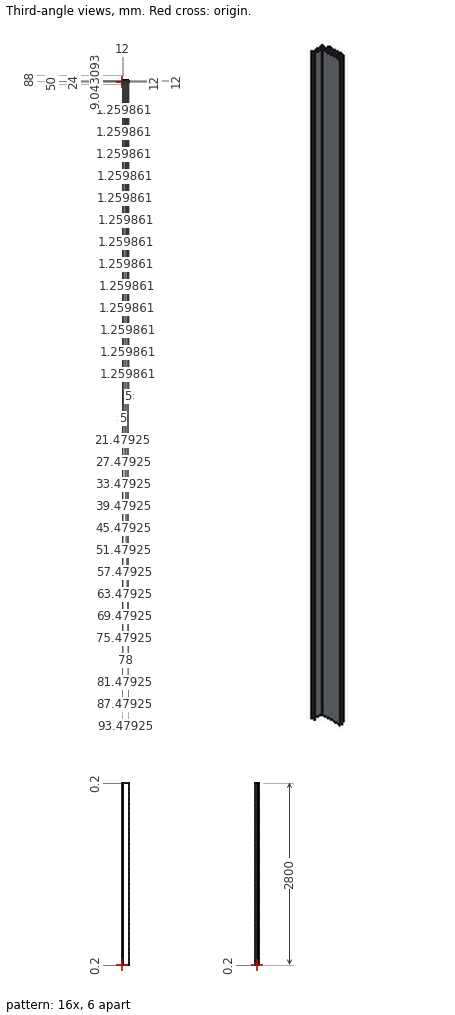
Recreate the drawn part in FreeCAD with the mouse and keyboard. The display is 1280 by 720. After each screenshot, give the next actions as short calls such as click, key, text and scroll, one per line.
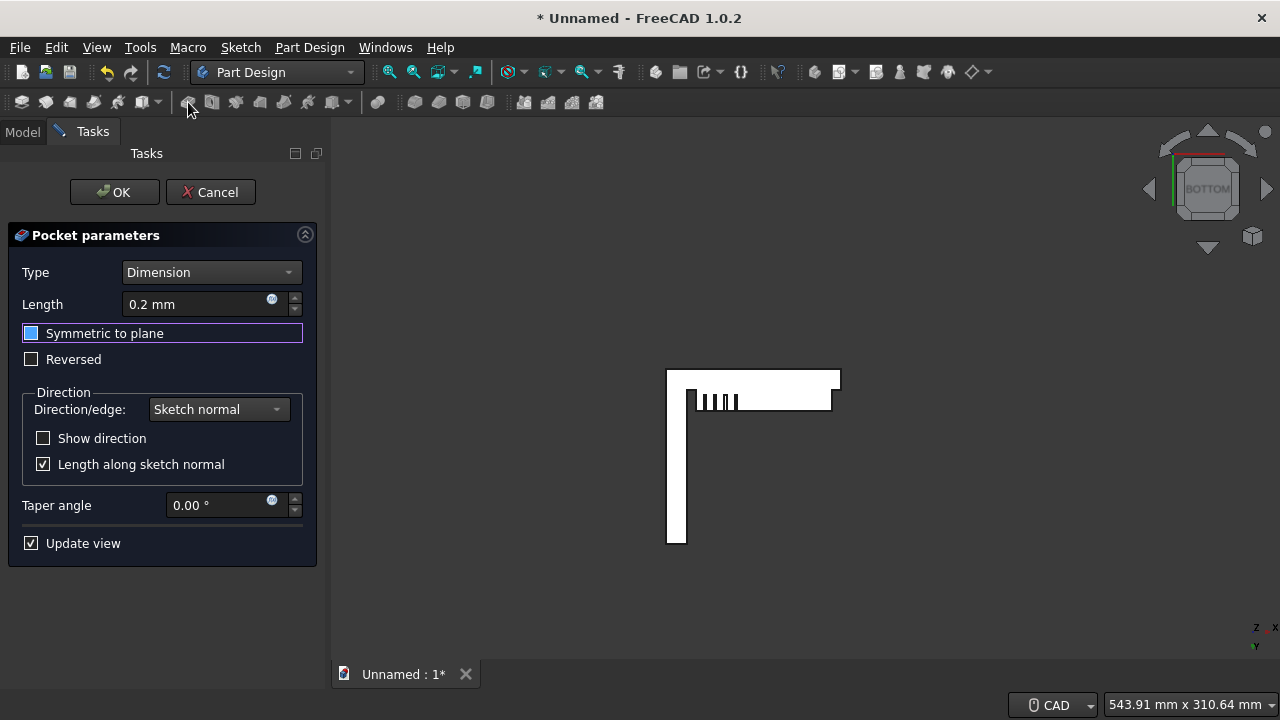
click(115, 192)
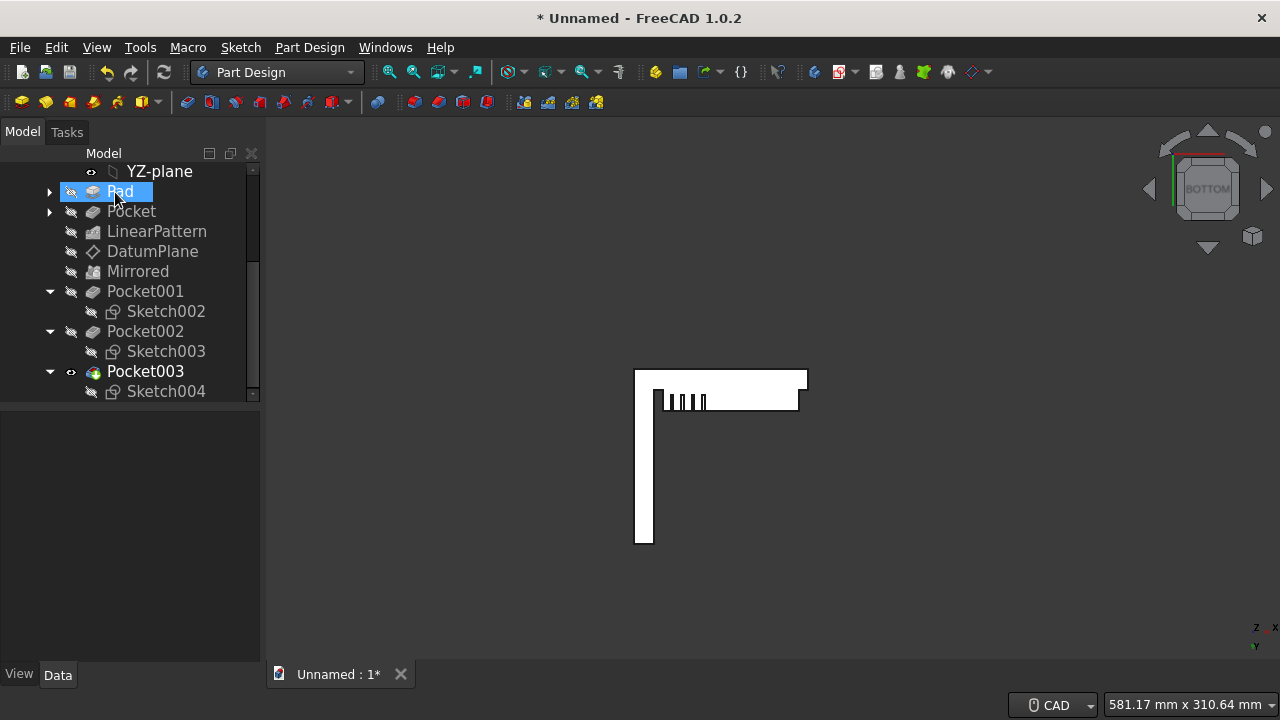
click(390, 72)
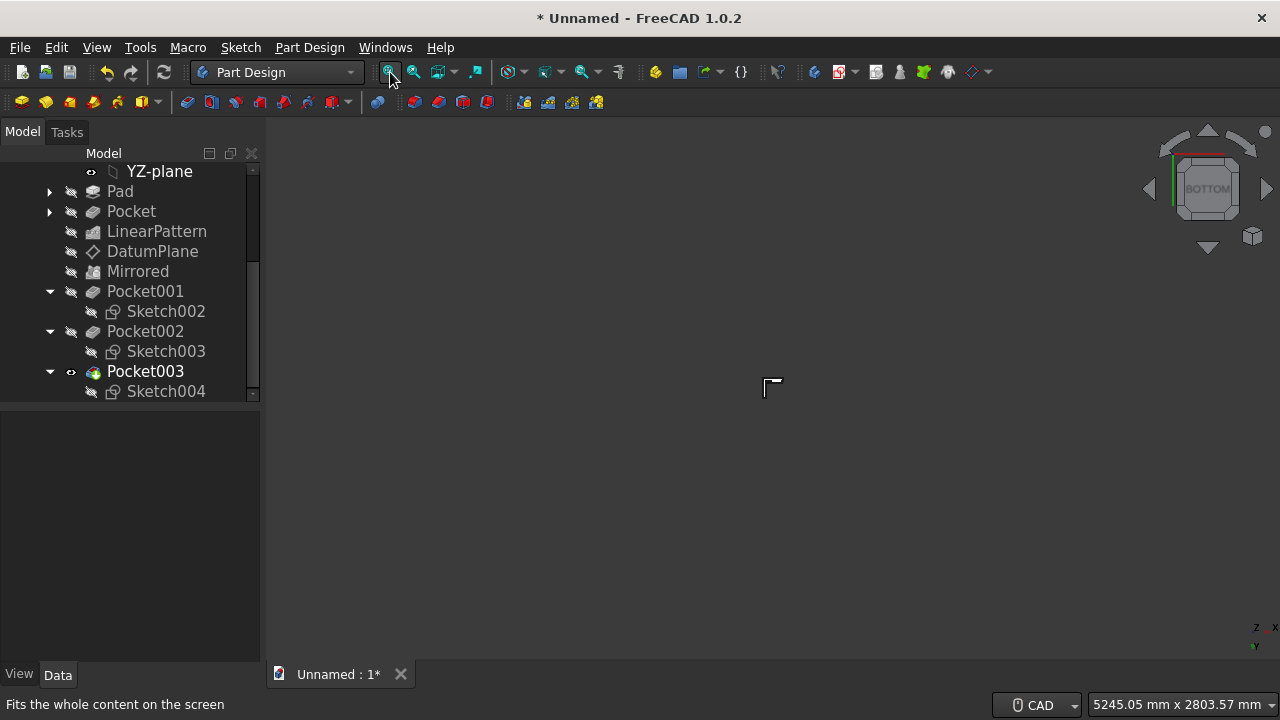
click(840, 72)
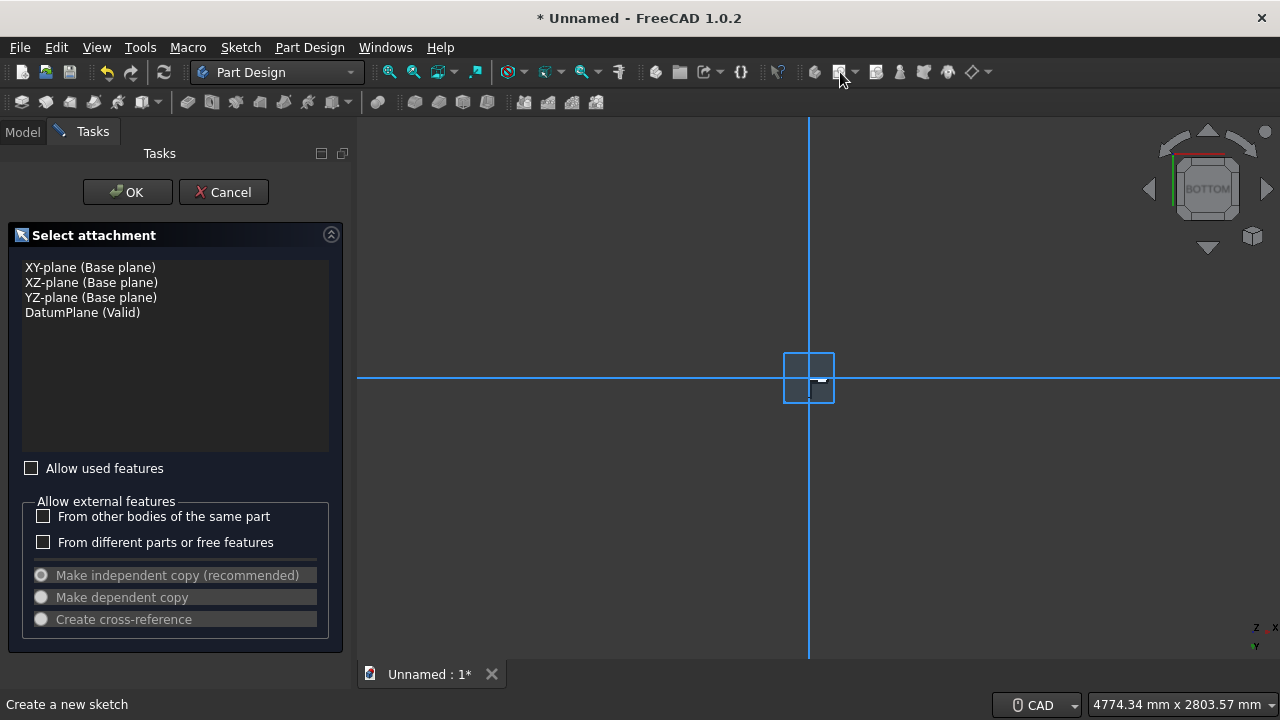
click(82, 268)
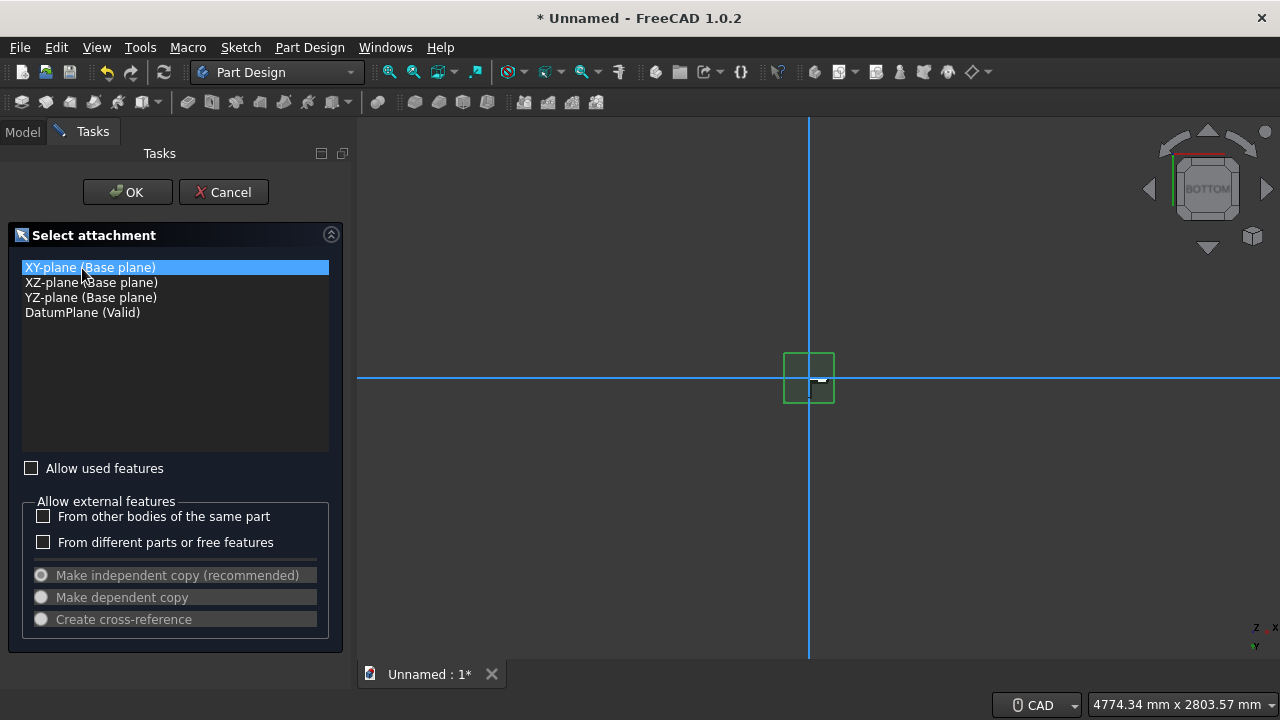
click(128, 192)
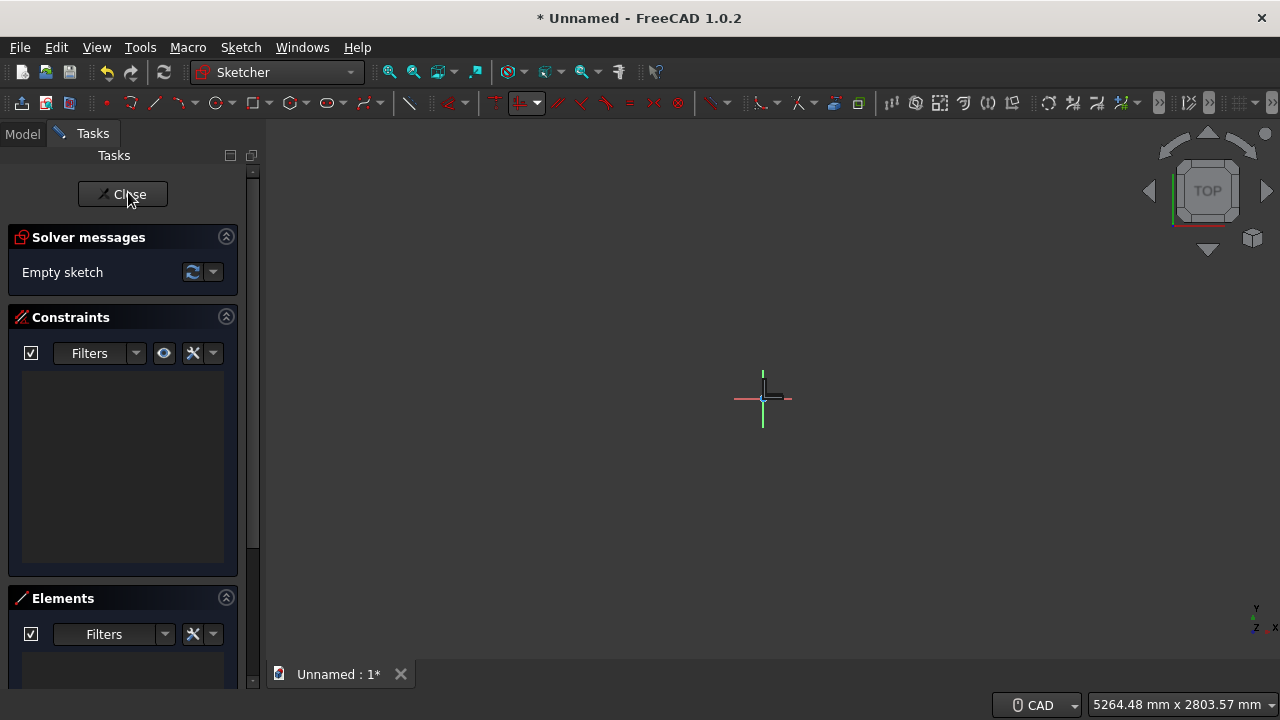
click(70, 104)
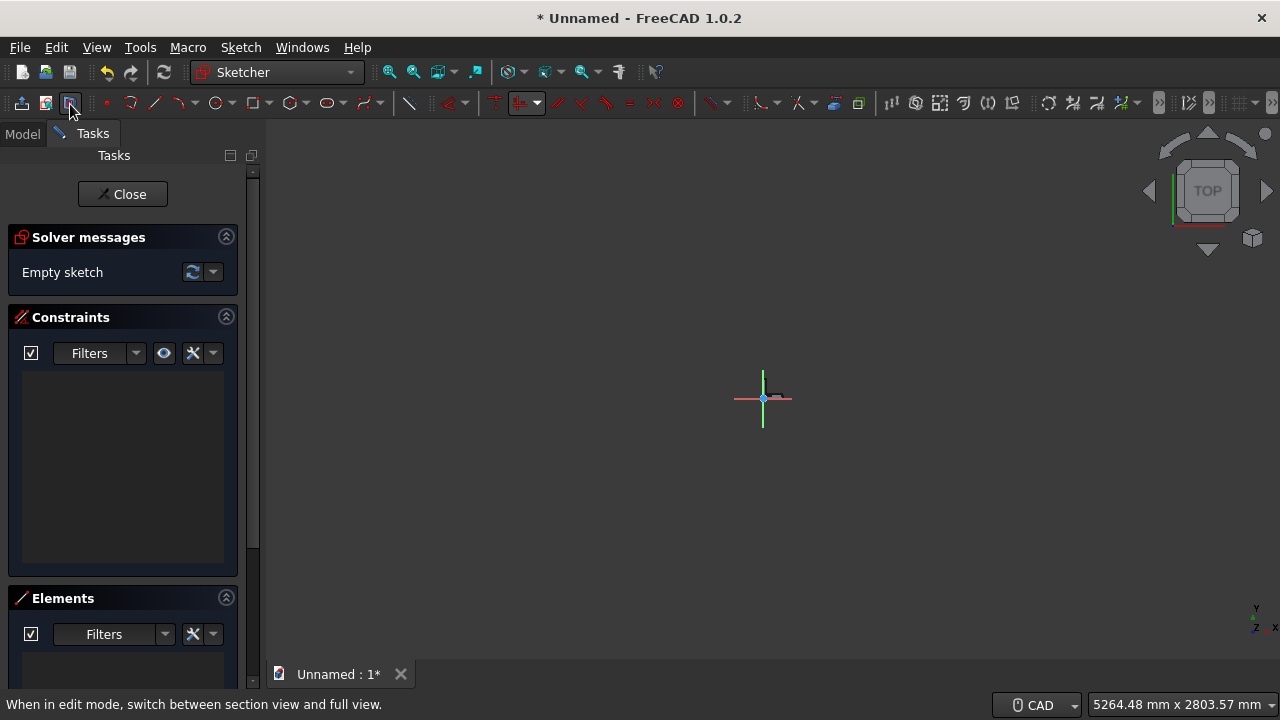
scroll(776, 395, up, 15)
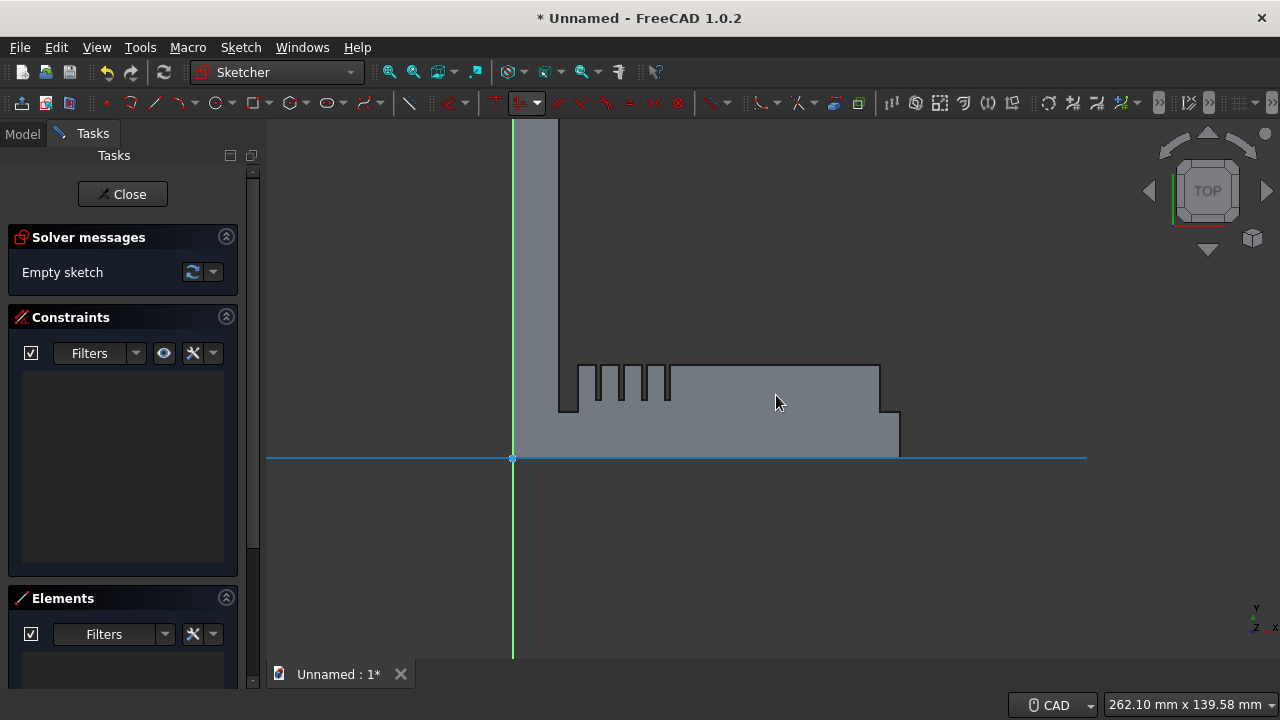
scroll(689, 382, up, 11)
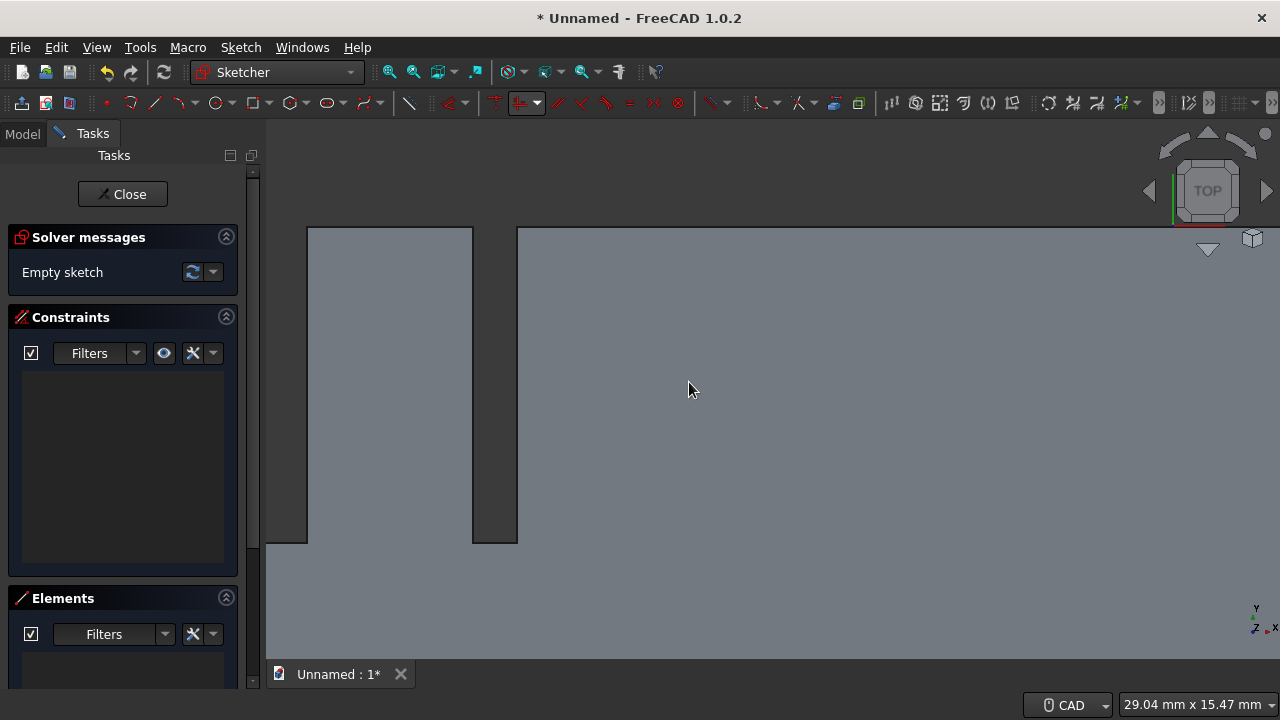
click(254, 104)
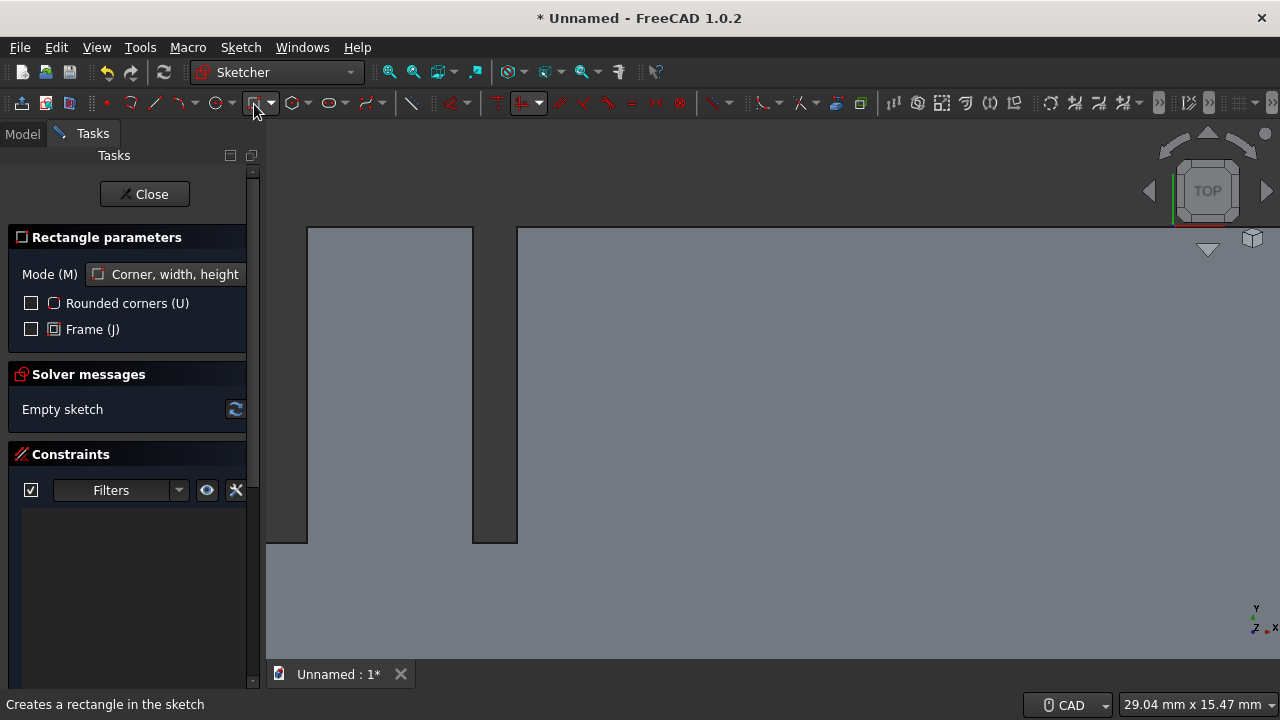
click(682, 227)
move(726, 543)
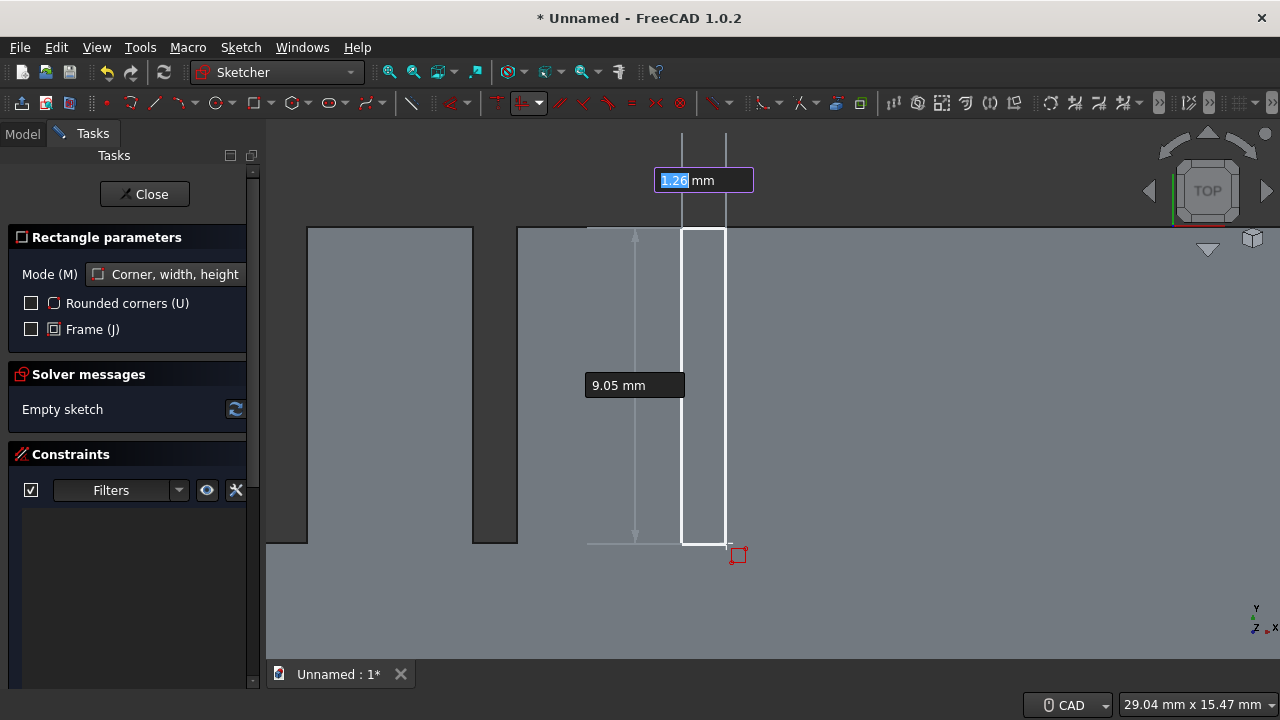
text(1.259861)
key(Tab)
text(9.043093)
key(Return)
key(Escape)